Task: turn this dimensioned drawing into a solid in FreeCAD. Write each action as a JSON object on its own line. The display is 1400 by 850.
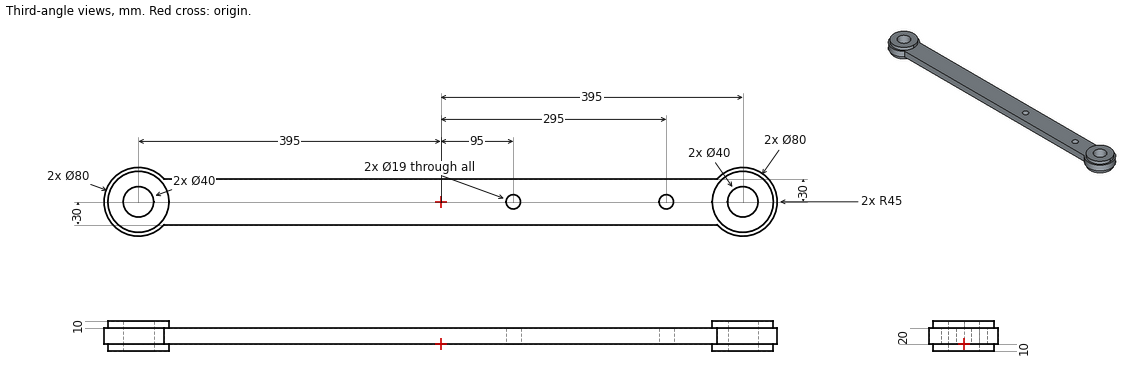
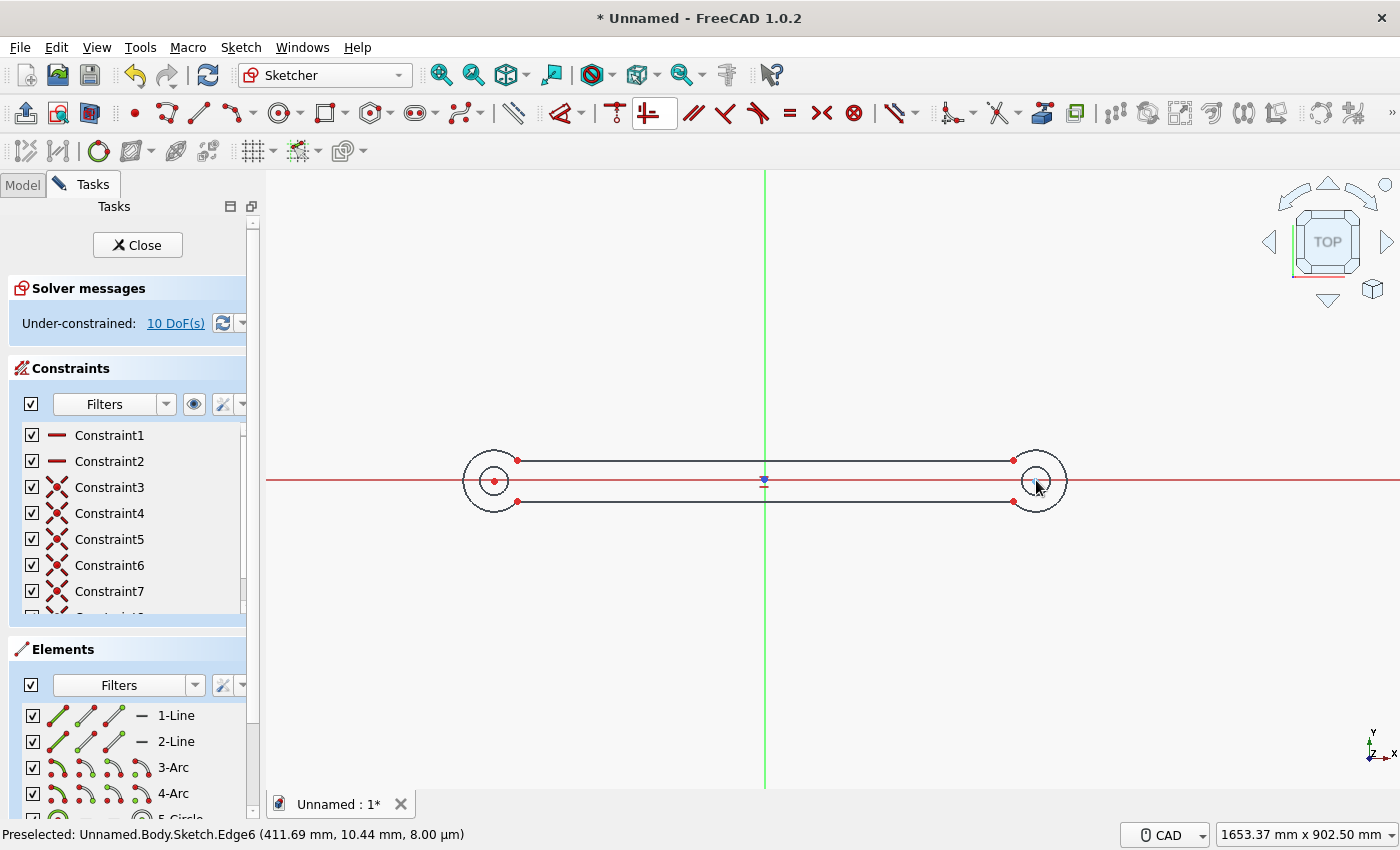
{"action": "left_click", "coordinate": [477, 456]}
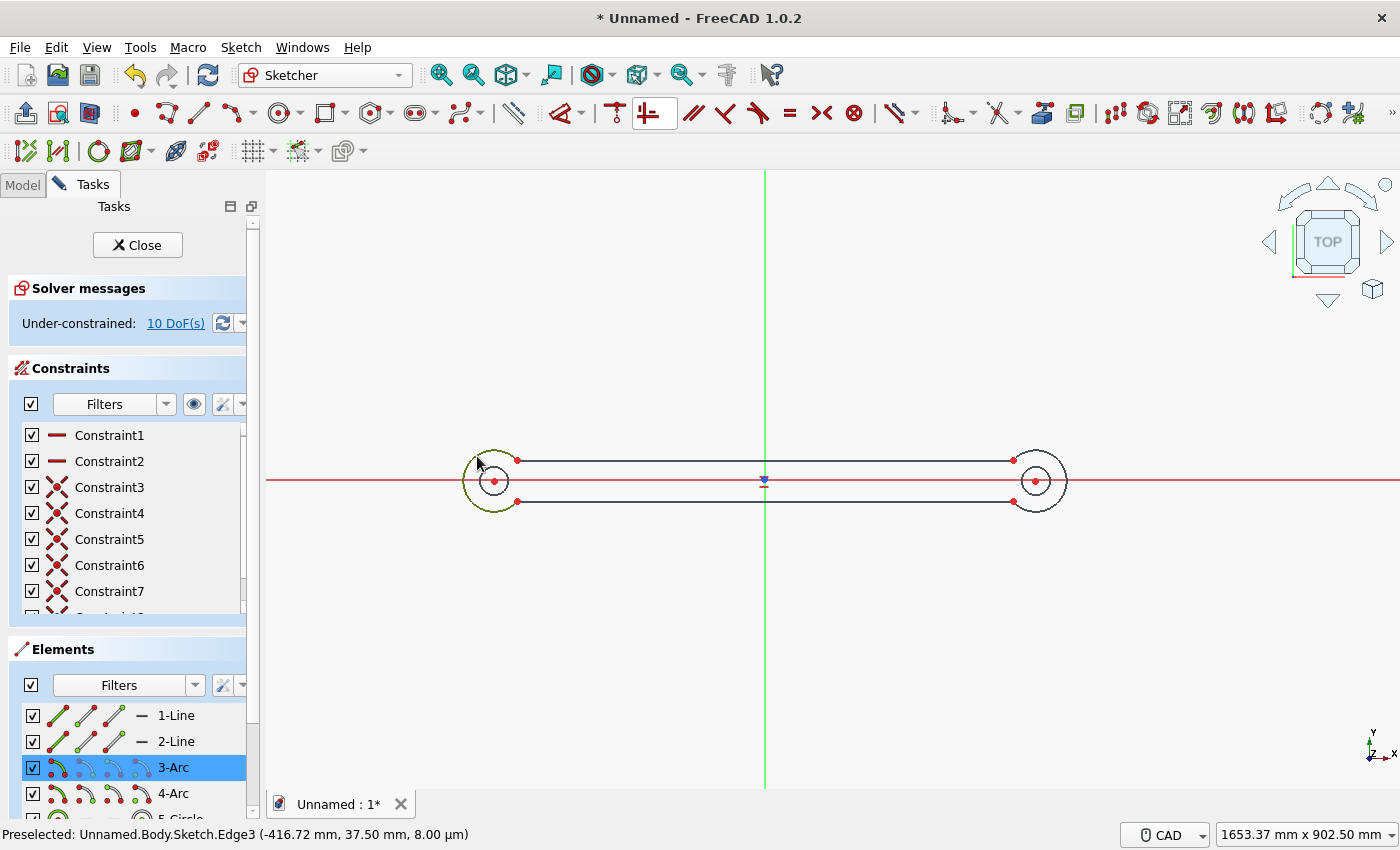
{"action": "left_click", "coordinate": [1053, 506]}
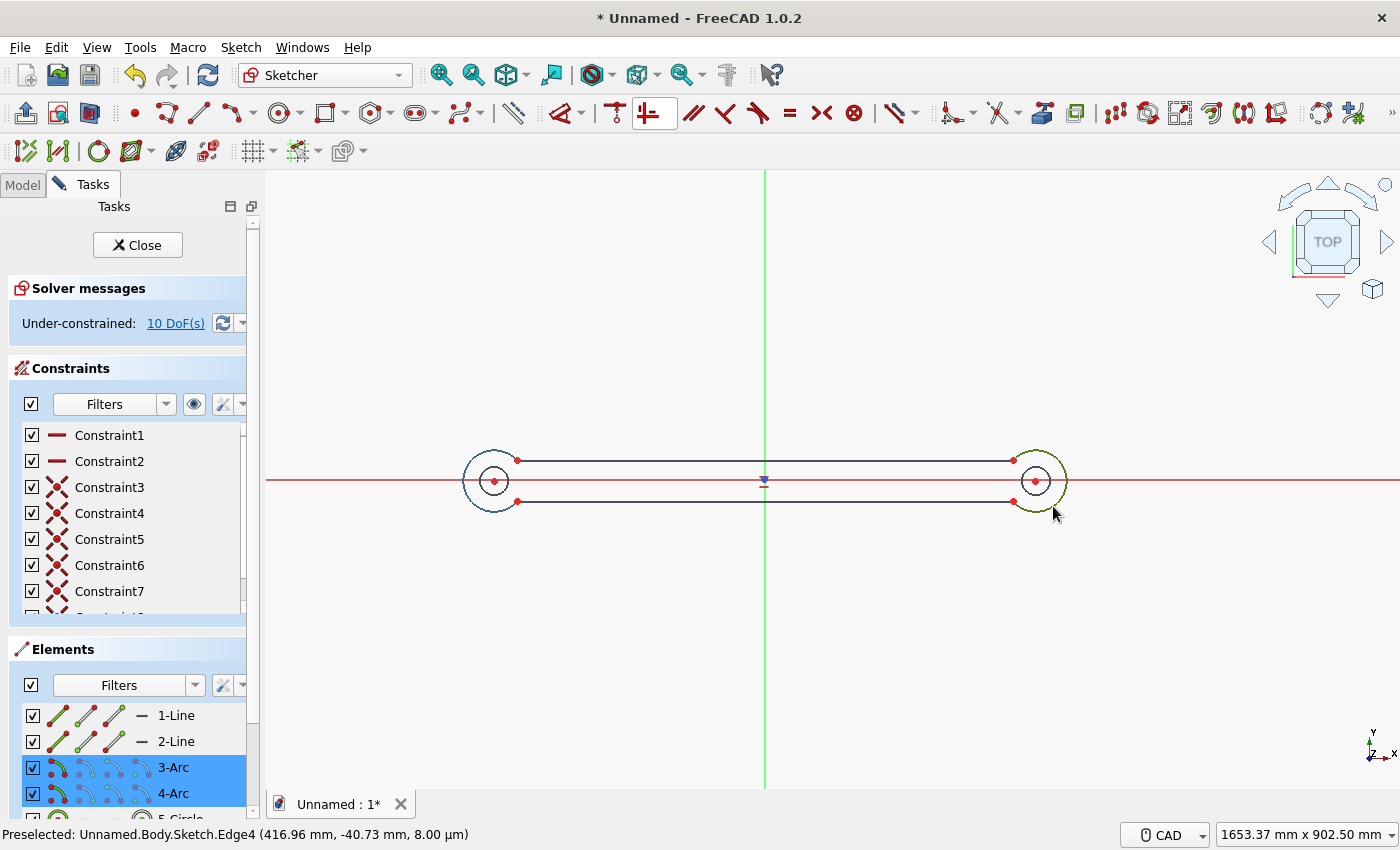
{"action": "left_click", "coordinate": [790, 114]}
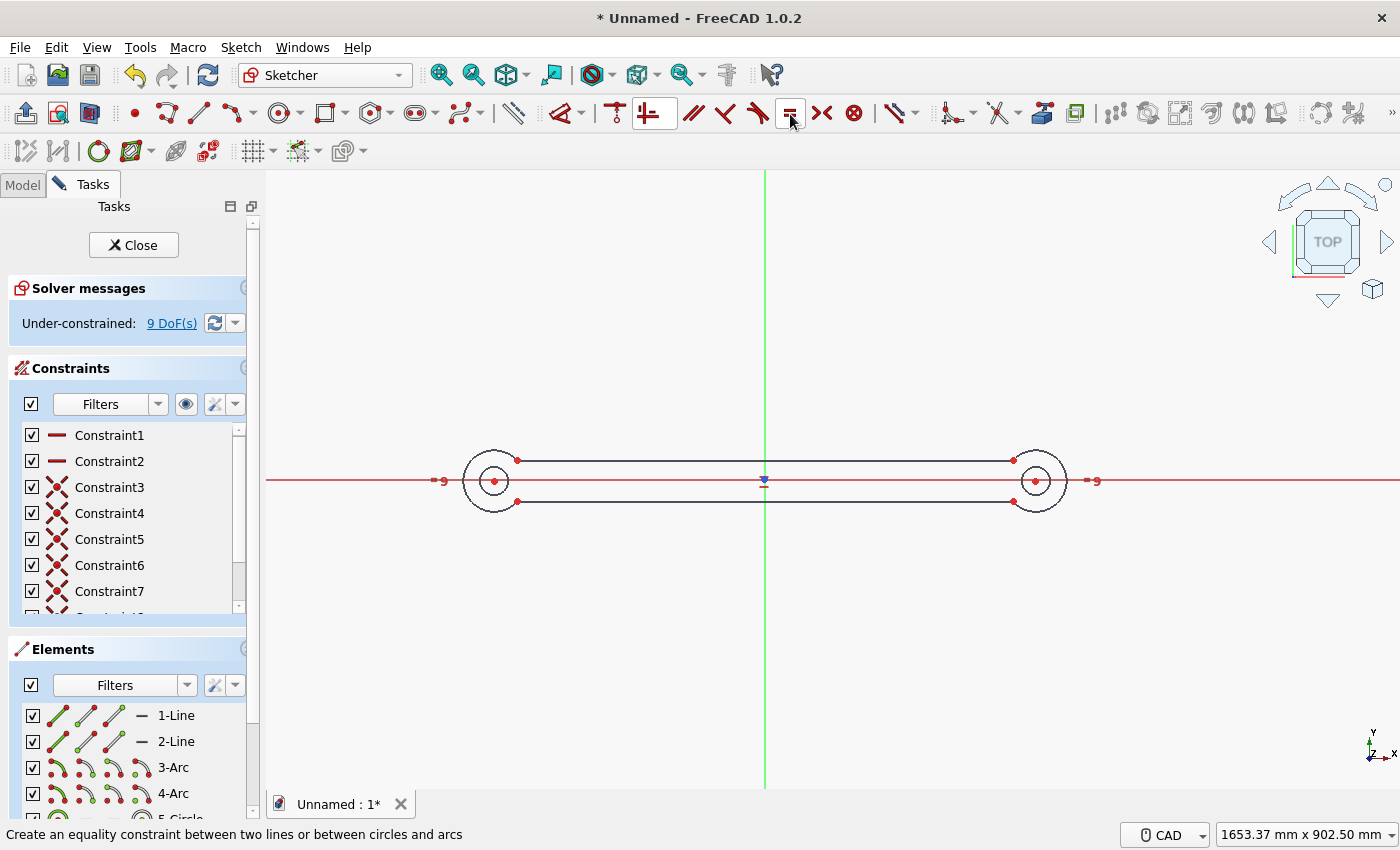
{"action": "scroll", "coordinate": [484, 491], "scroll_direction": "up", "scroll_amount": 2}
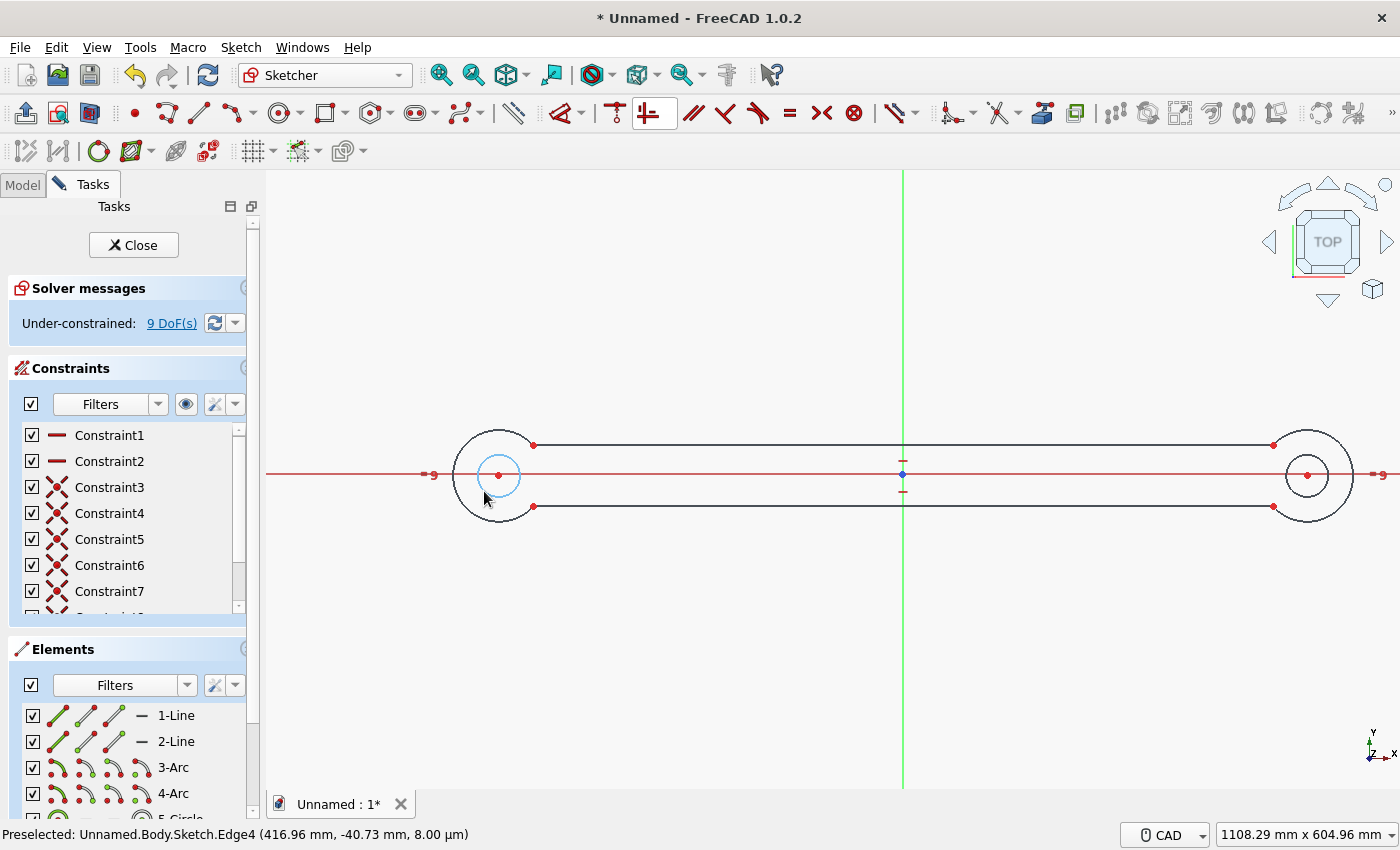
{"action": "left_click", "coordinate": [484, 491]}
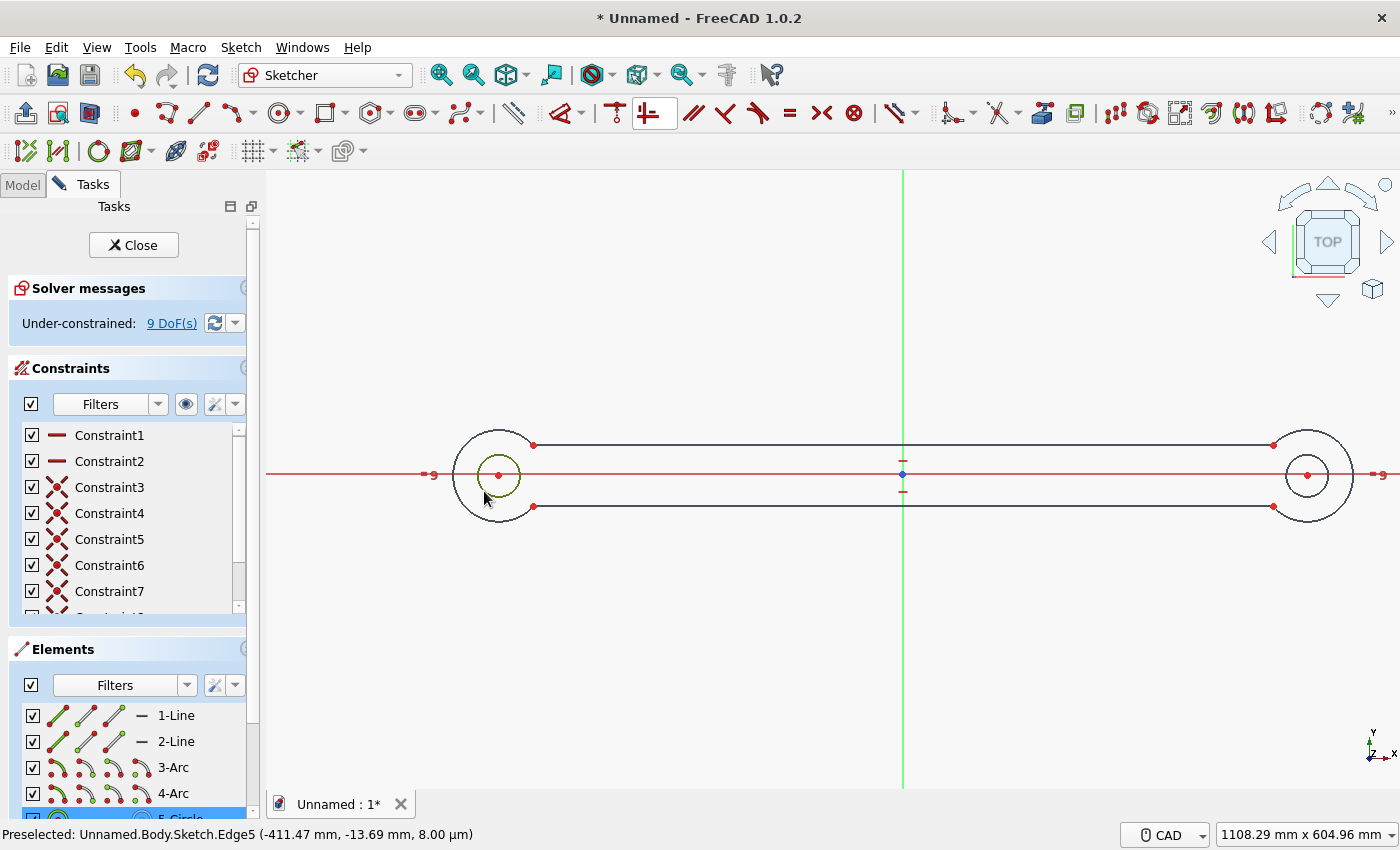
{"action": "scroll", "coordinate": [483, 490], "scroll_direction": "down", "scroll_amount": 2}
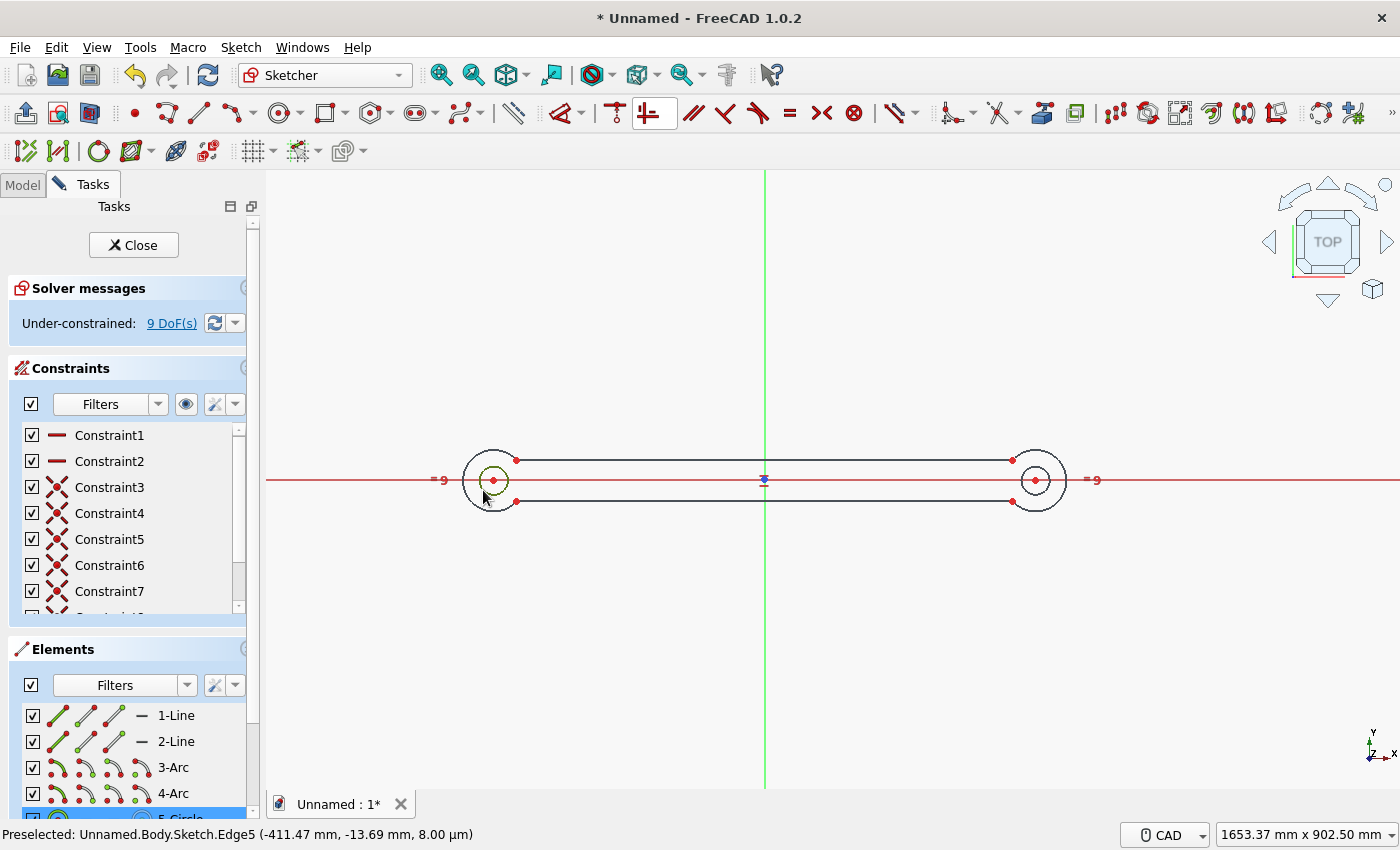
{"action": "scroll", "coordinate": [1045, 471], "scroll_direction": "up", "scroll_amount": 3}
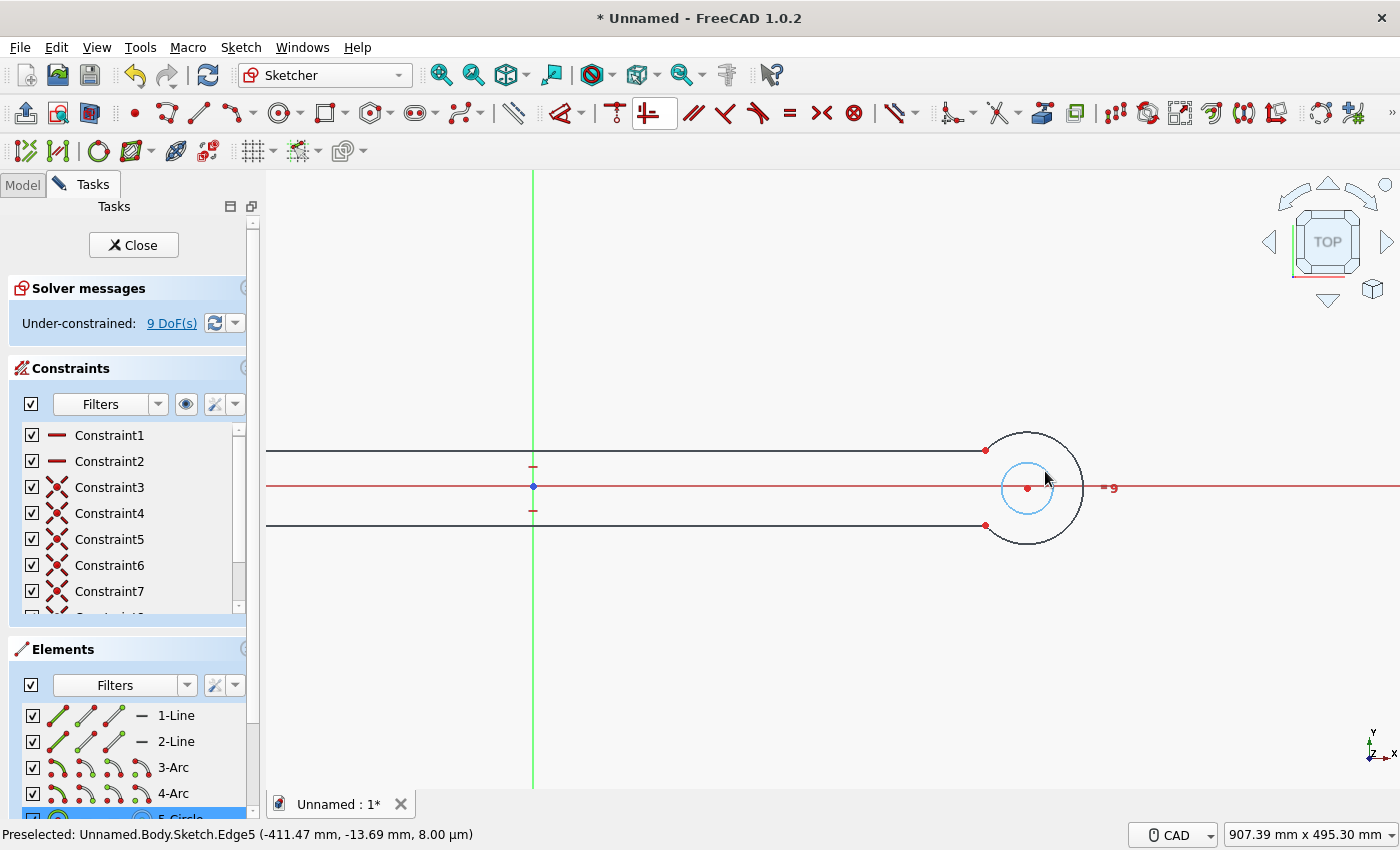
{"action": "left_click", "coordinate": [1045, 470]}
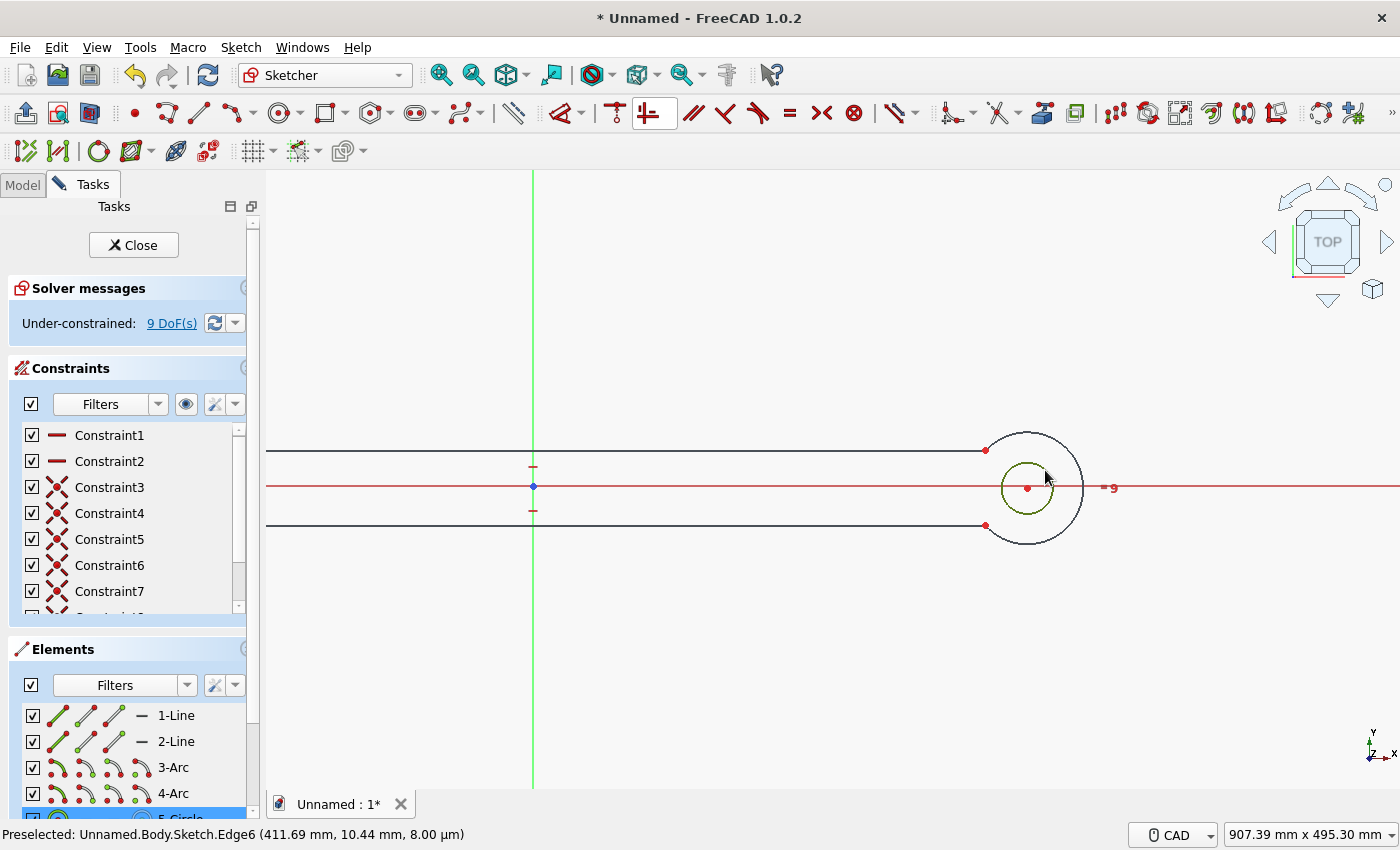
{"action": "left_click", "coordinate": [790, 114]}